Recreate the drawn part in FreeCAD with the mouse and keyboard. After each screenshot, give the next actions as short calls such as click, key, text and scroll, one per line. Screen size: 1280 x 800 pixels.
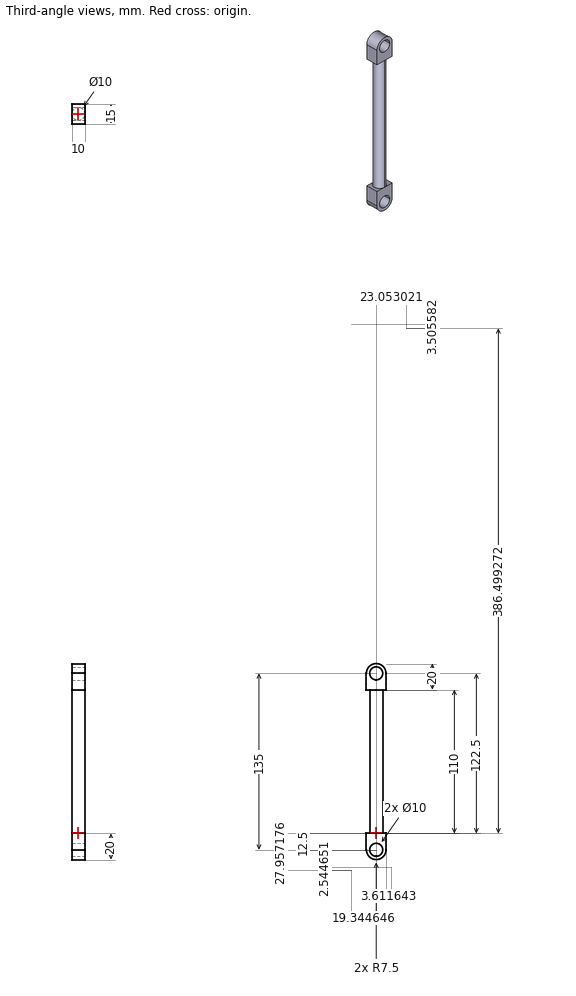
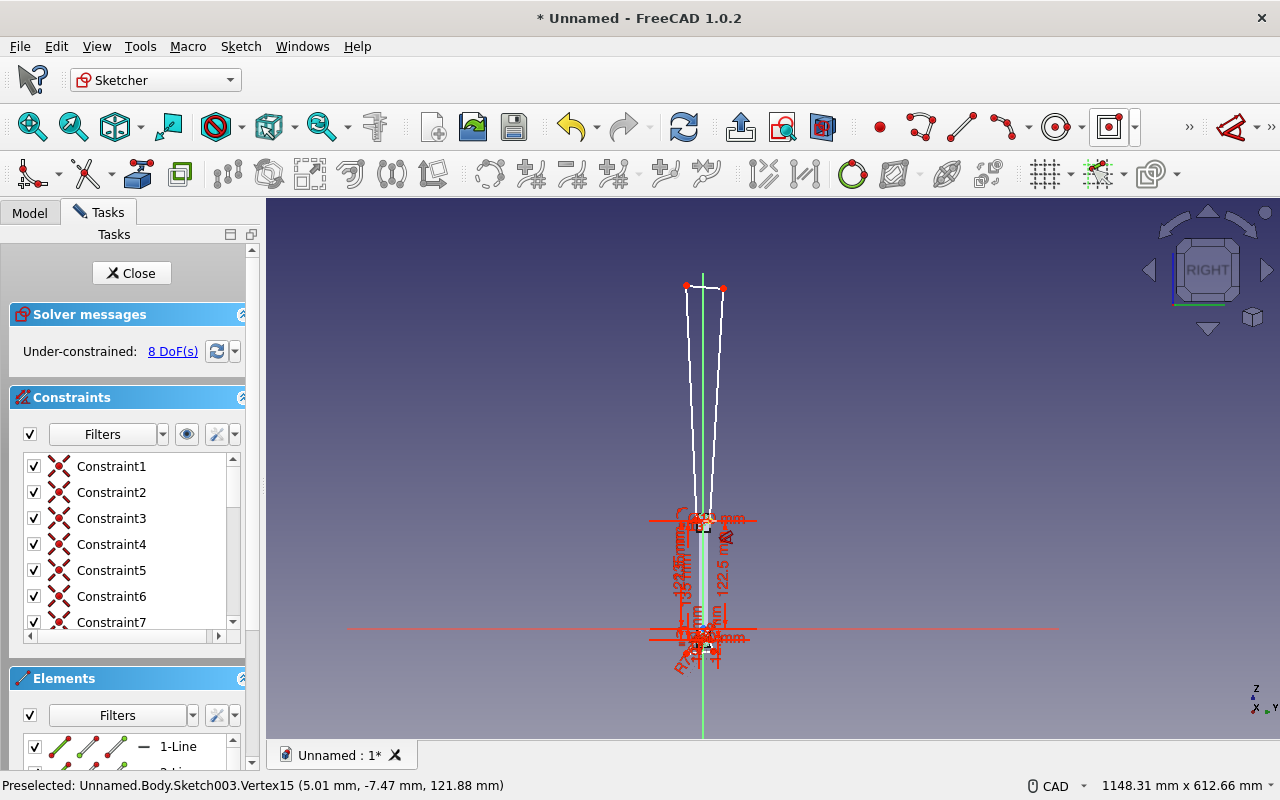
scroll(694, 653, up, 15)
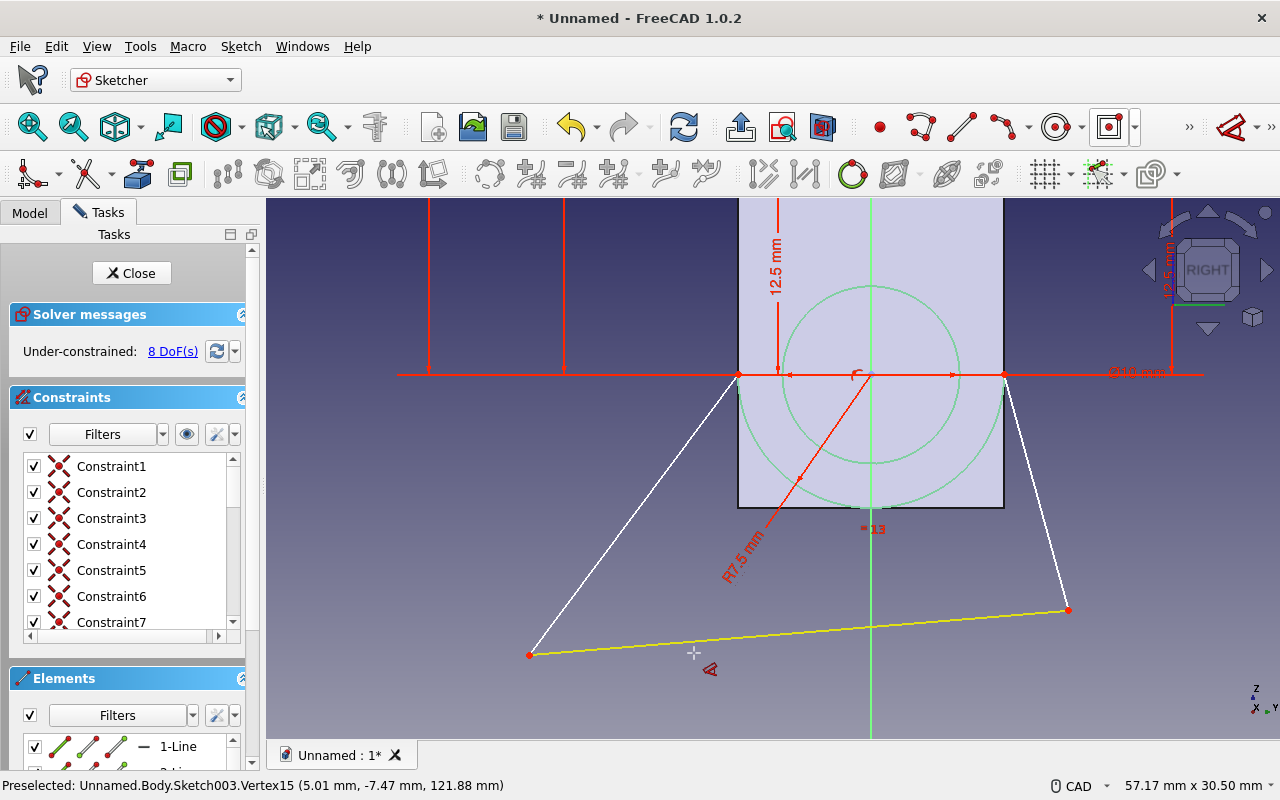
click(691, 642)
click(495, 633)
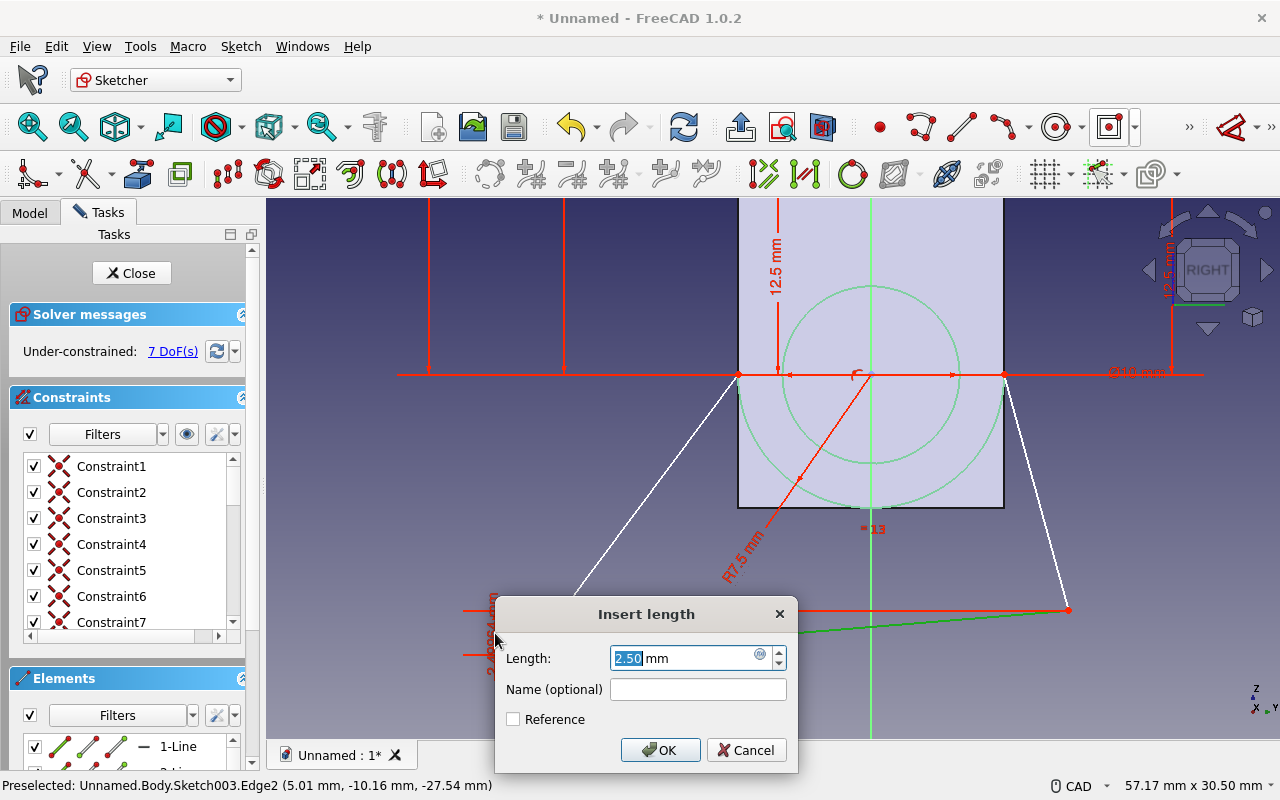
text(2.544651)
key(Return)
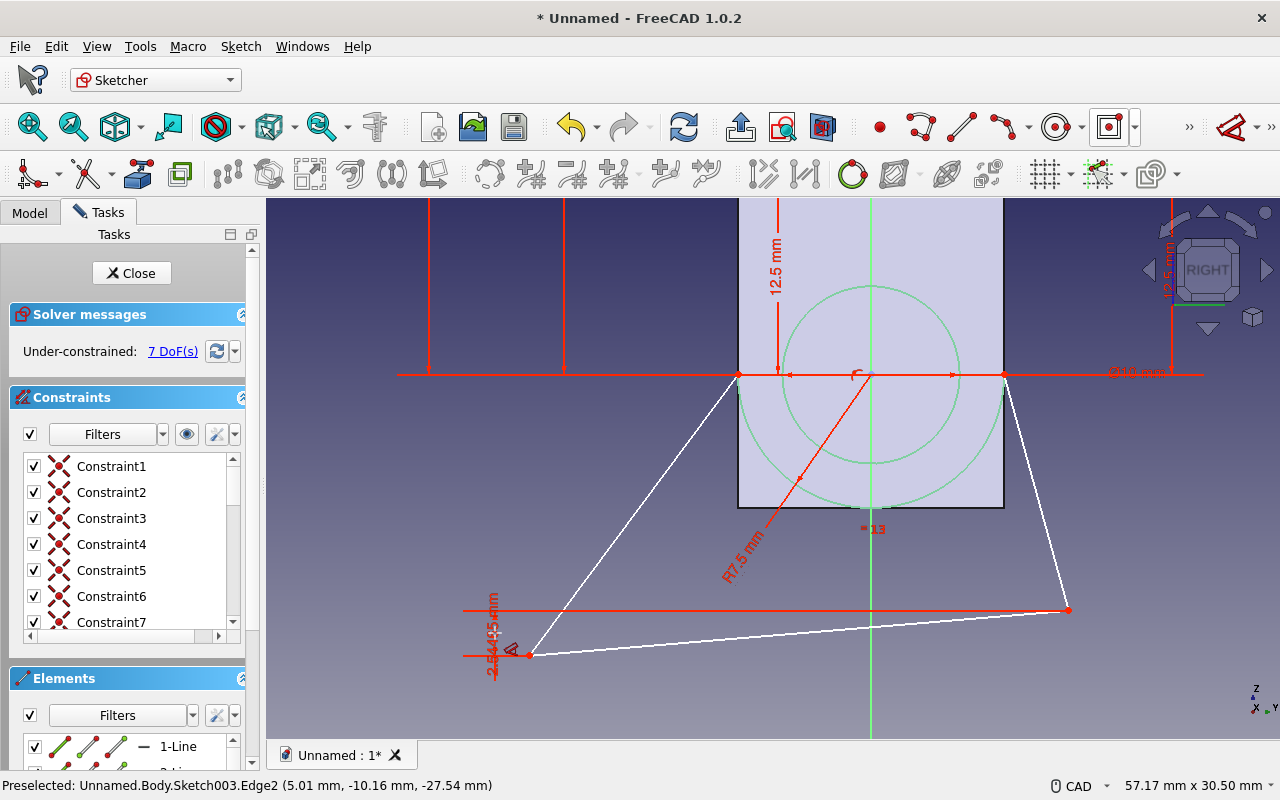
click(1049, 540)
click(1036, 645)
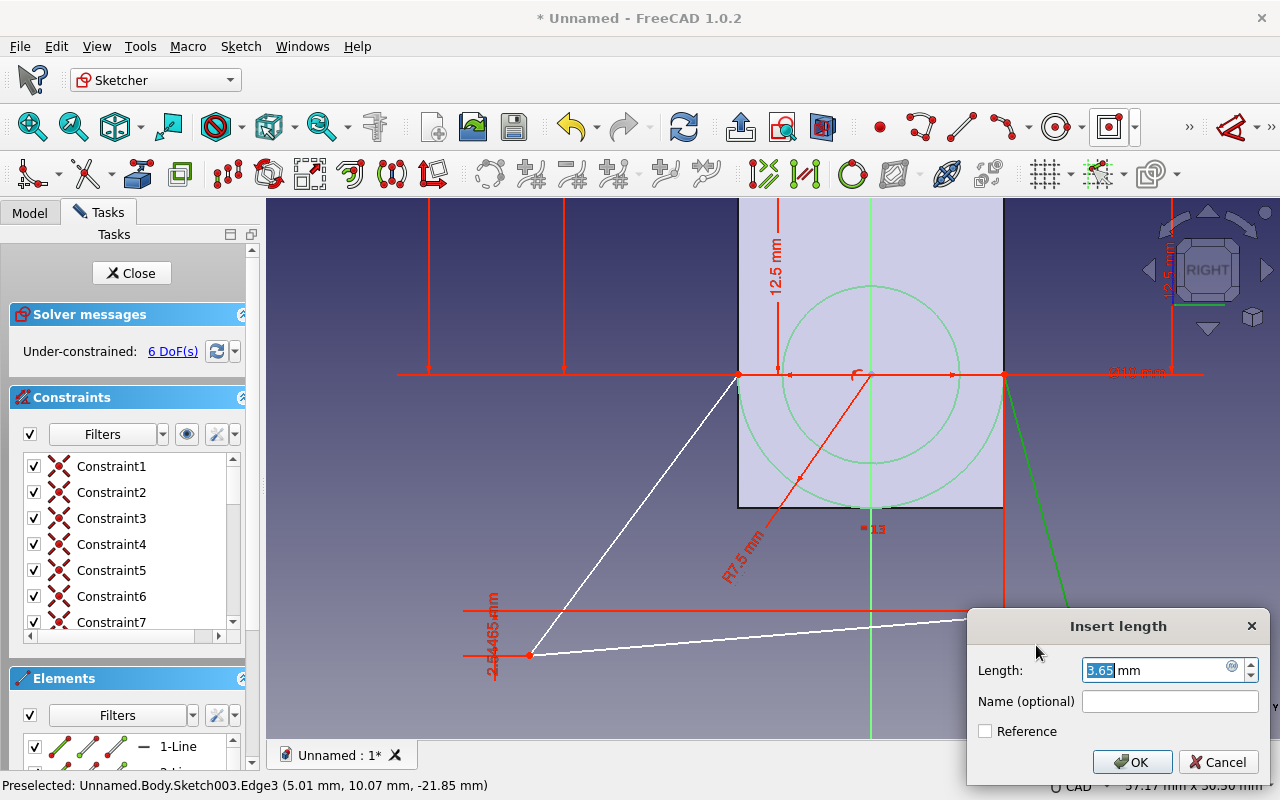
text(3.611643)
key(Return)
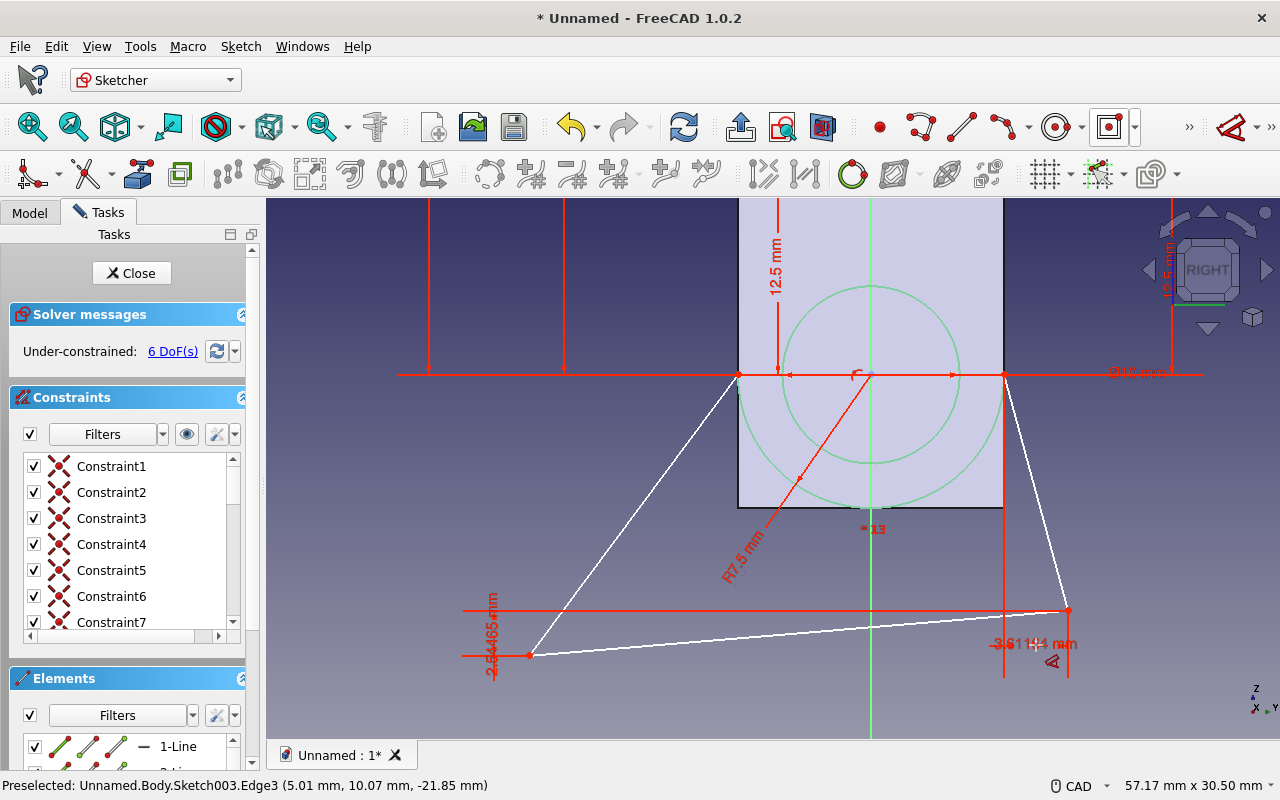
scroll(694, 653, down, 15)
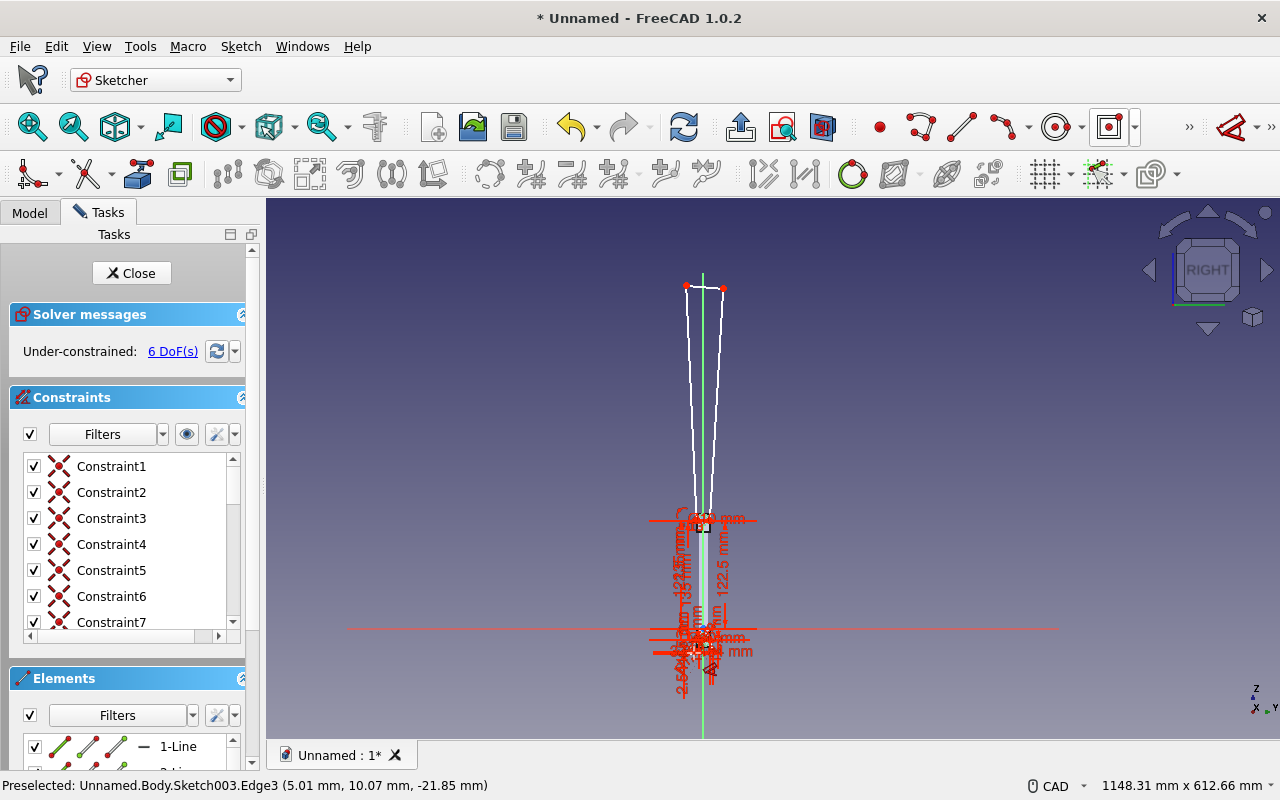
scroll(712, 288, up, 13)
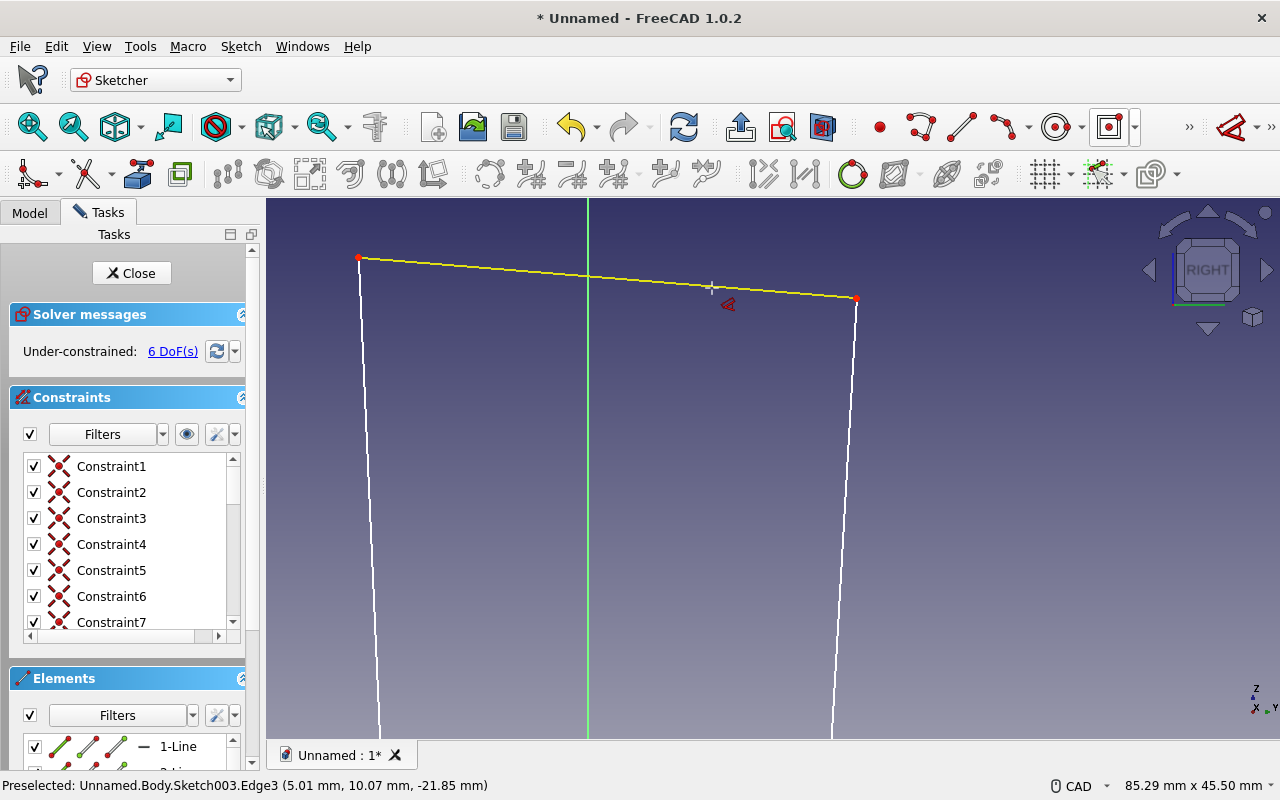
click(707, 286)
click(325, 278)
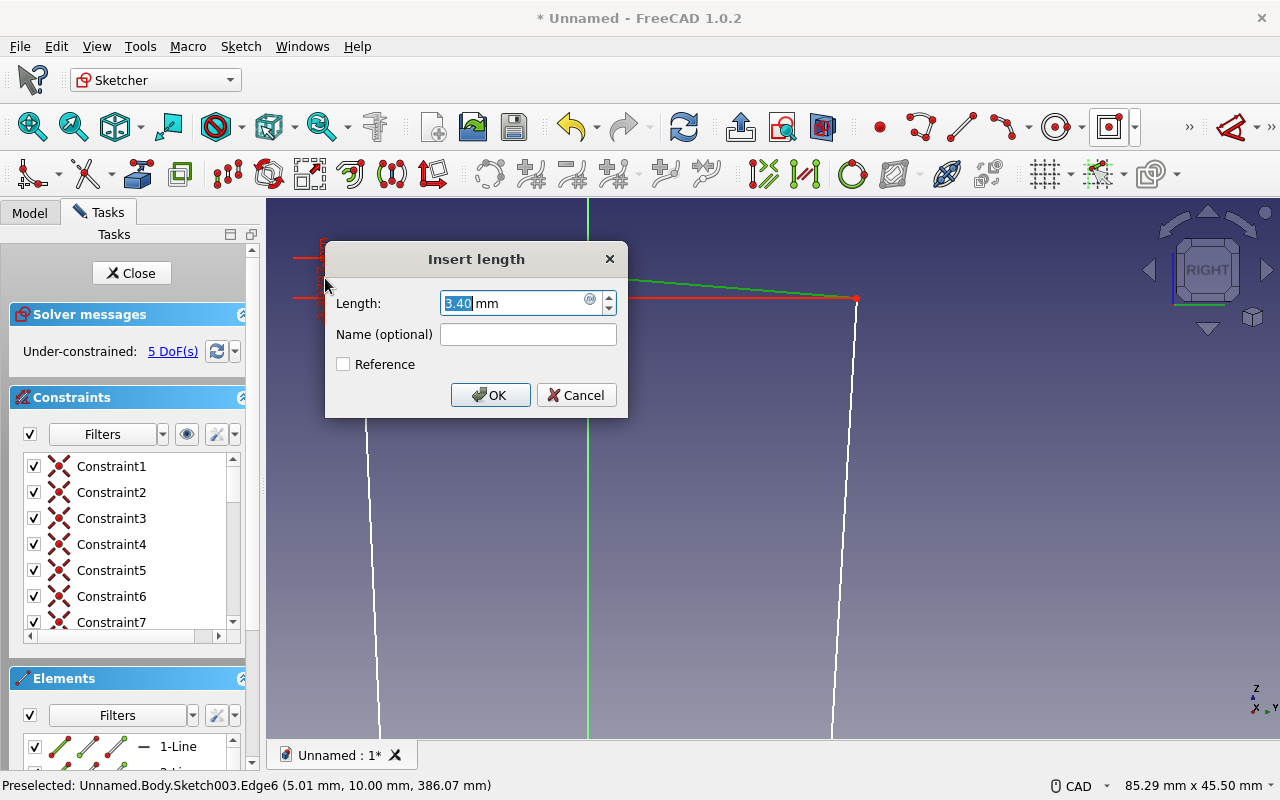
text(3.505582)
key(Return)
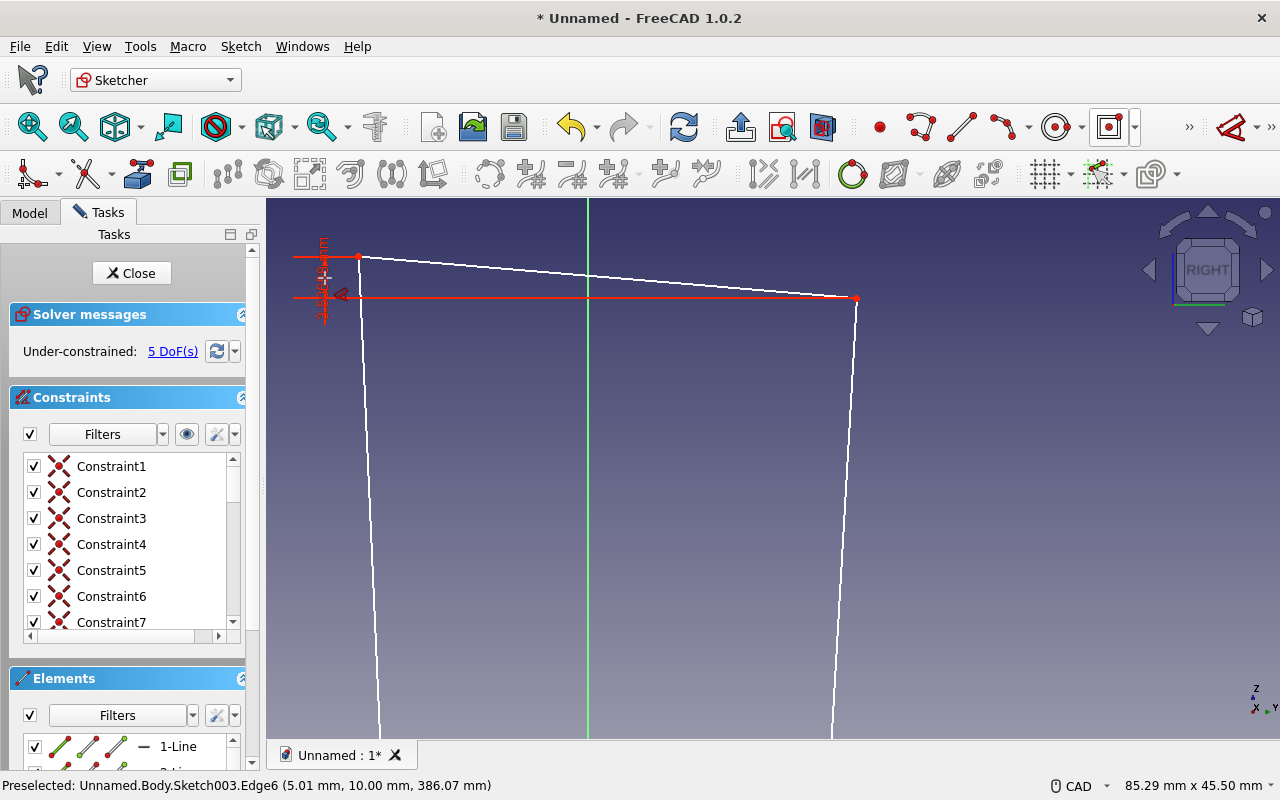
scroll(712, 288, down, 13)